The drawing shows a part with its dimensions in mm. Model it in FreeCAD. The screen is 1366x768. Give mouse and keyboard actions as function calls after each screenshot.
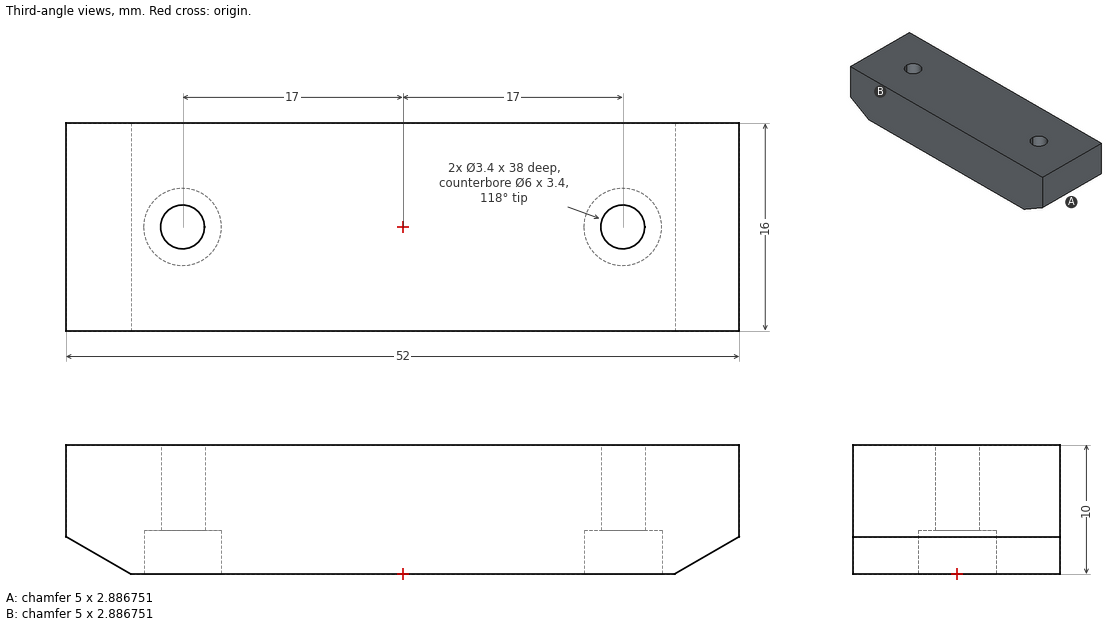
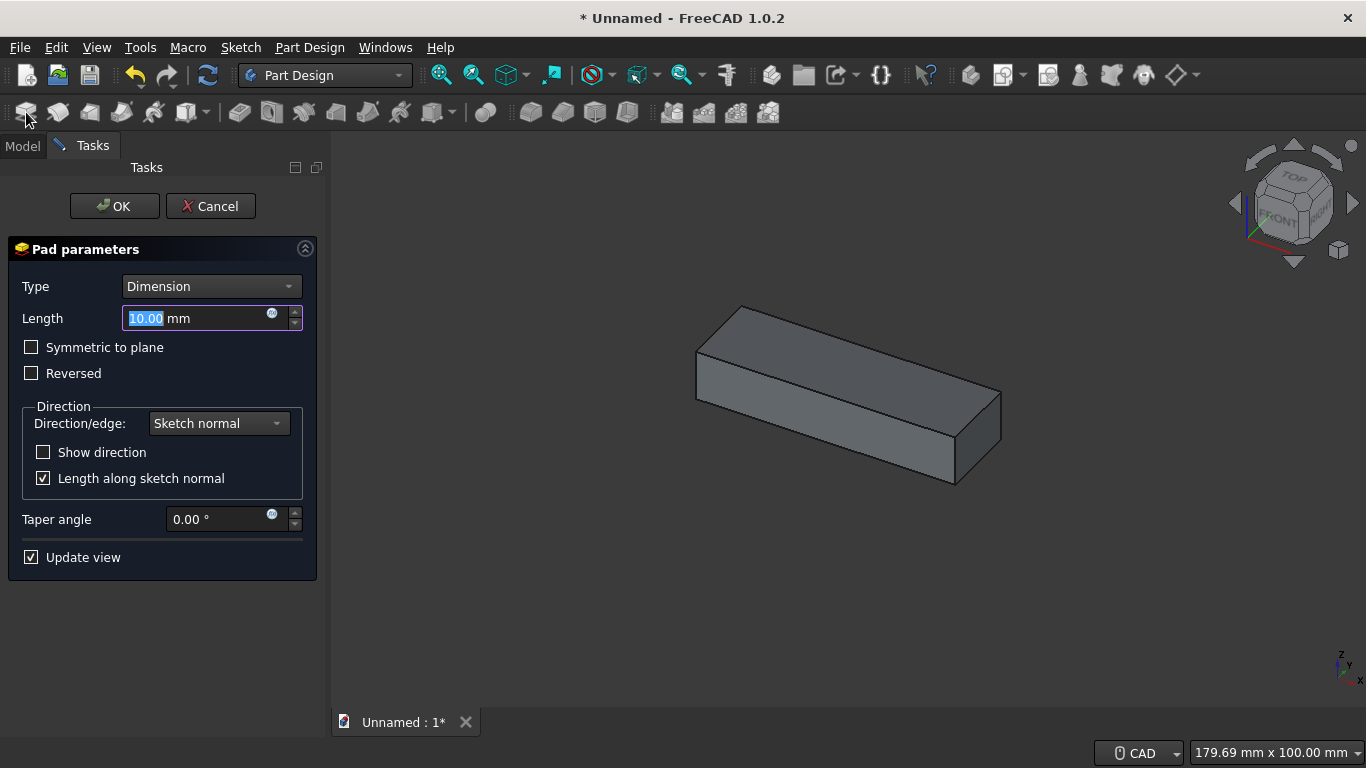
text(10)
key(Tab)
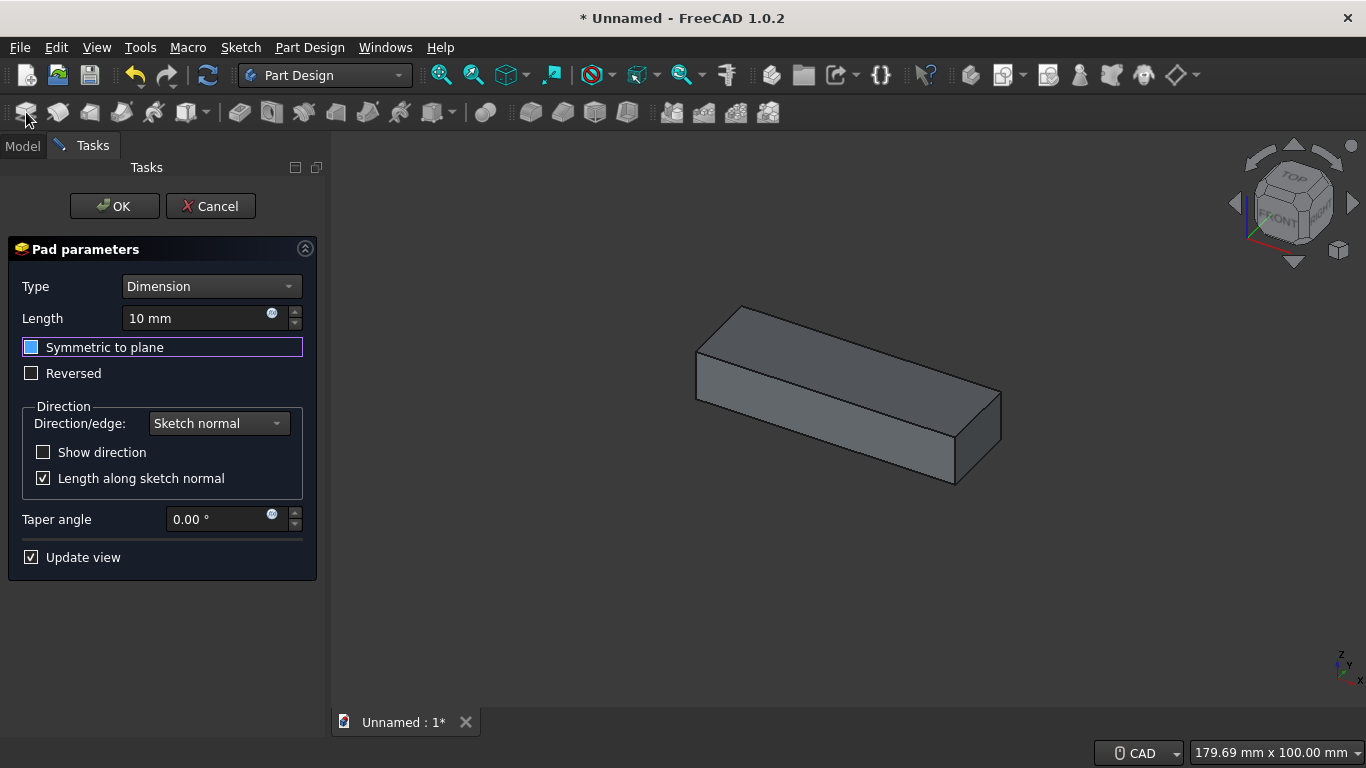
click(115, 206)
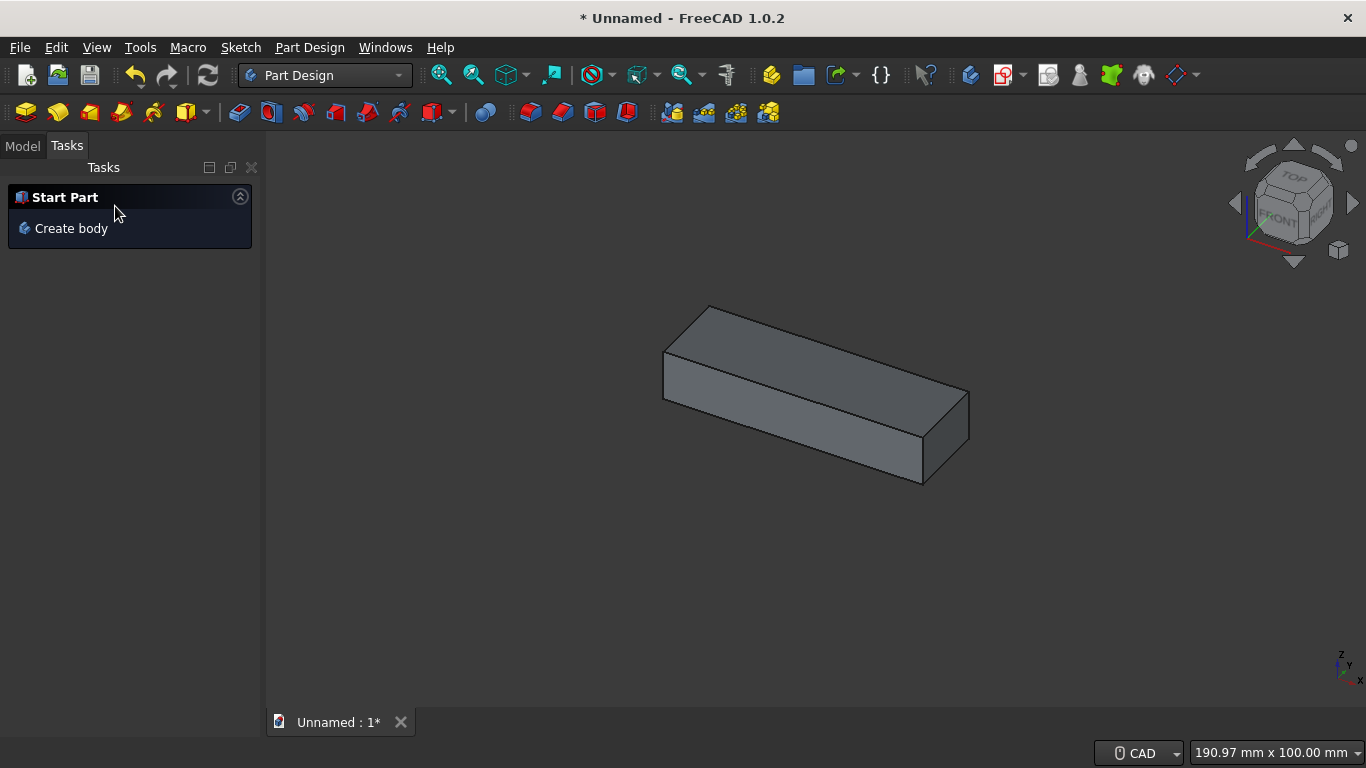
click(442, 76)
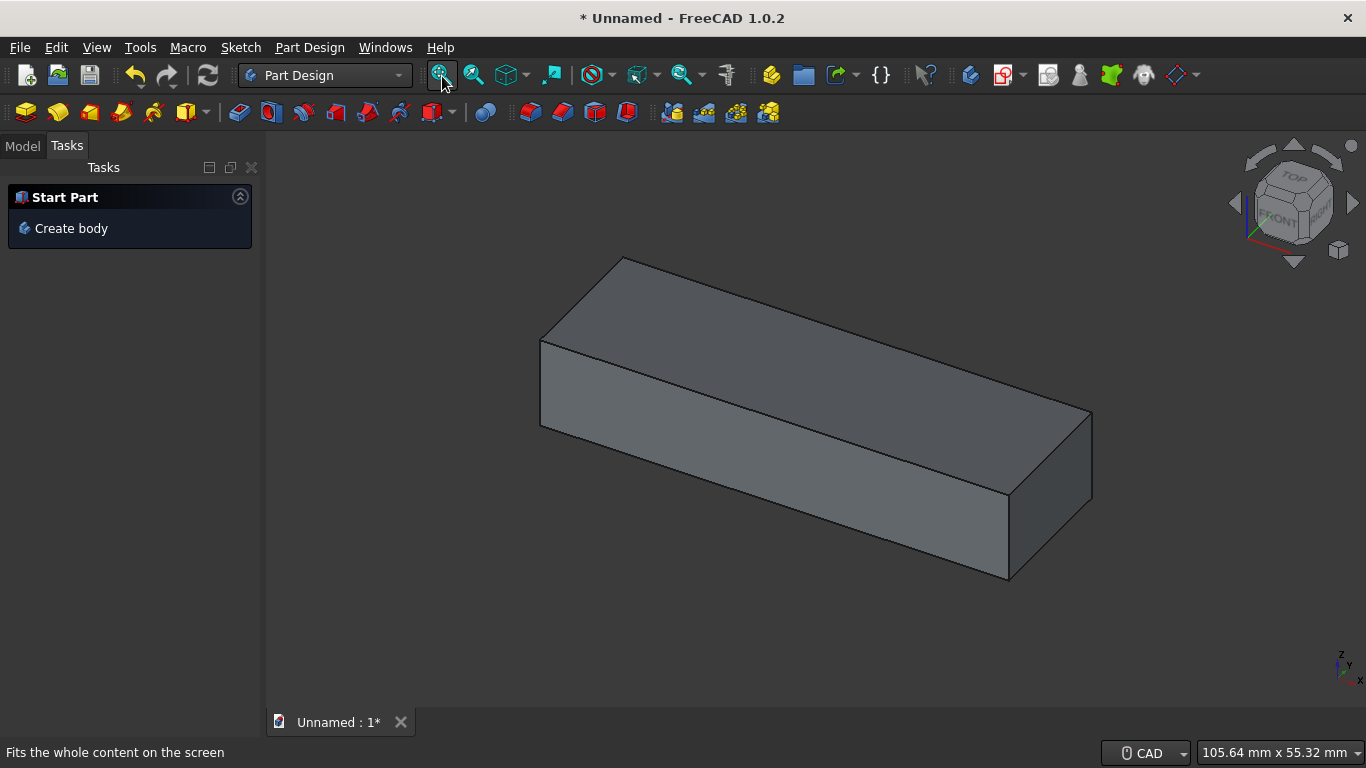
key(5)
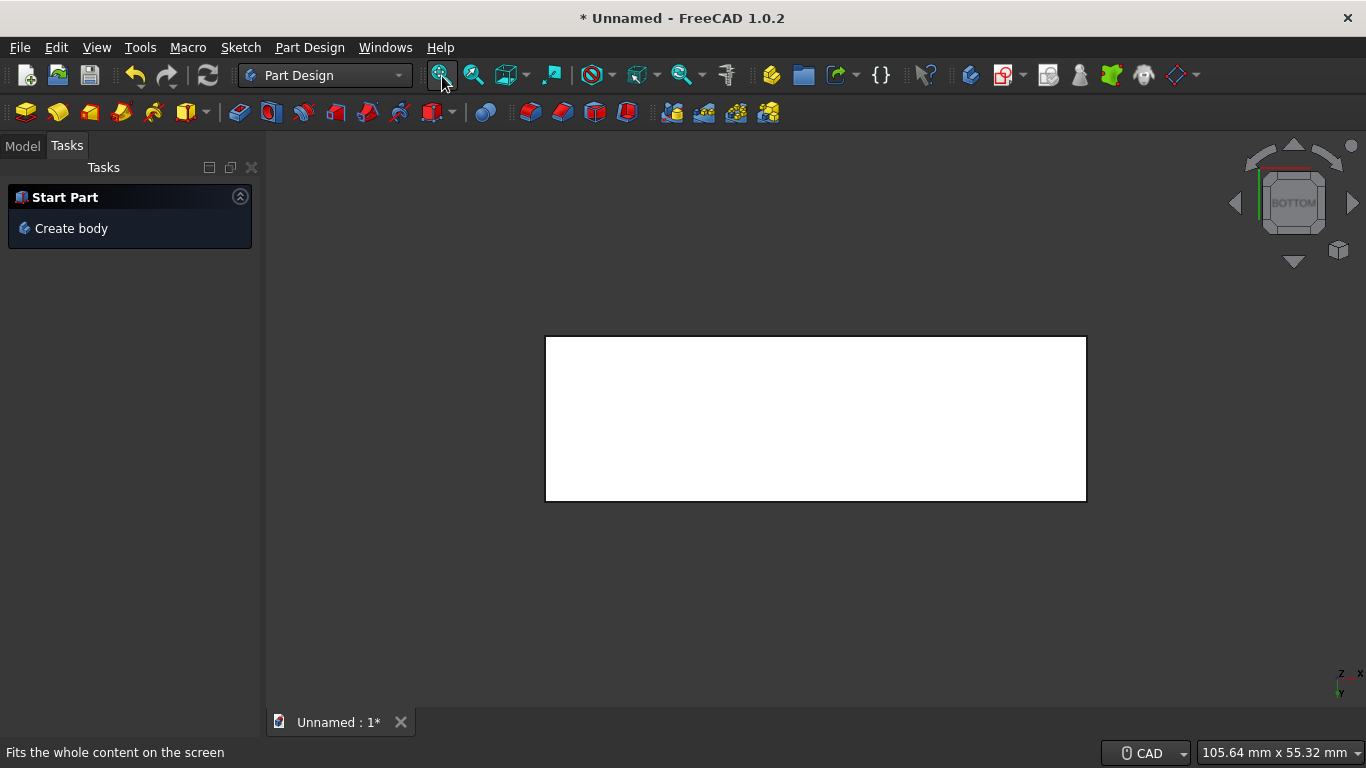
click(971, 418)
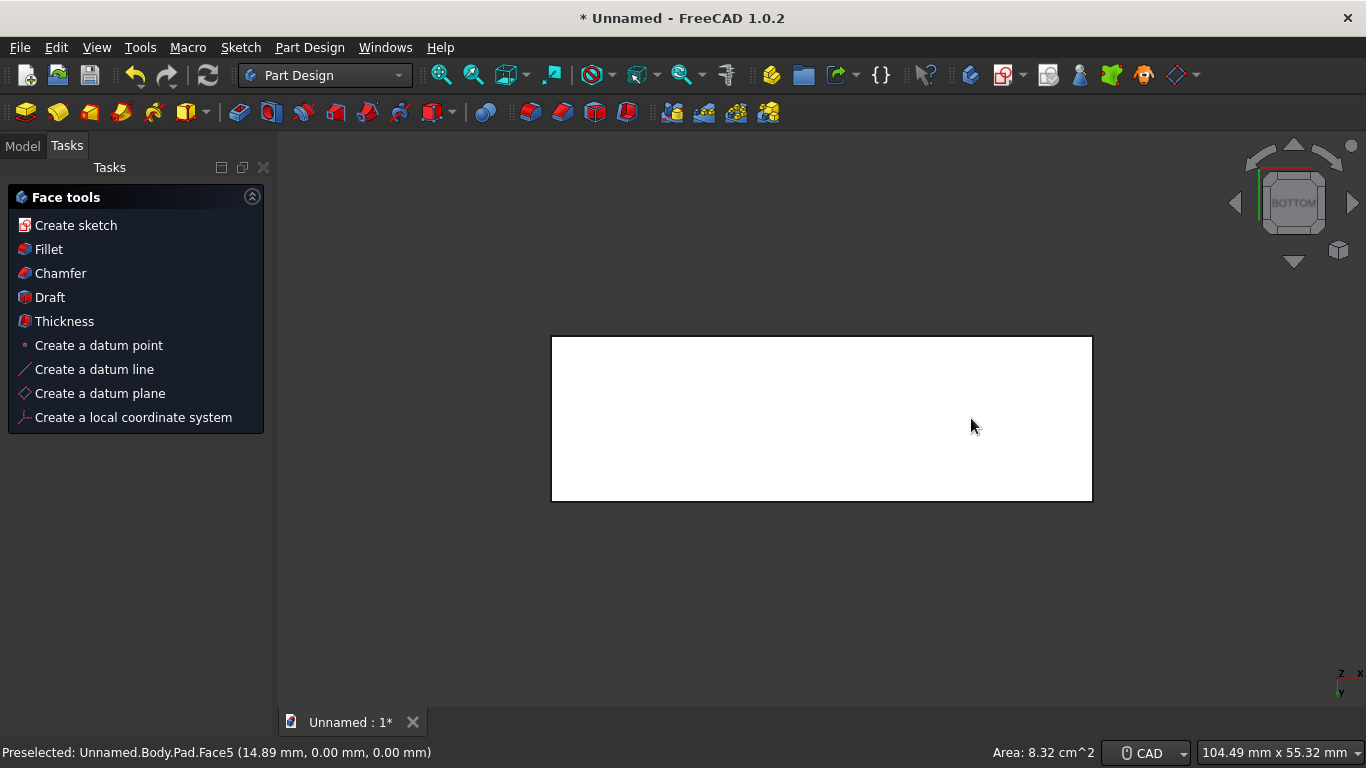
click(1004, 76)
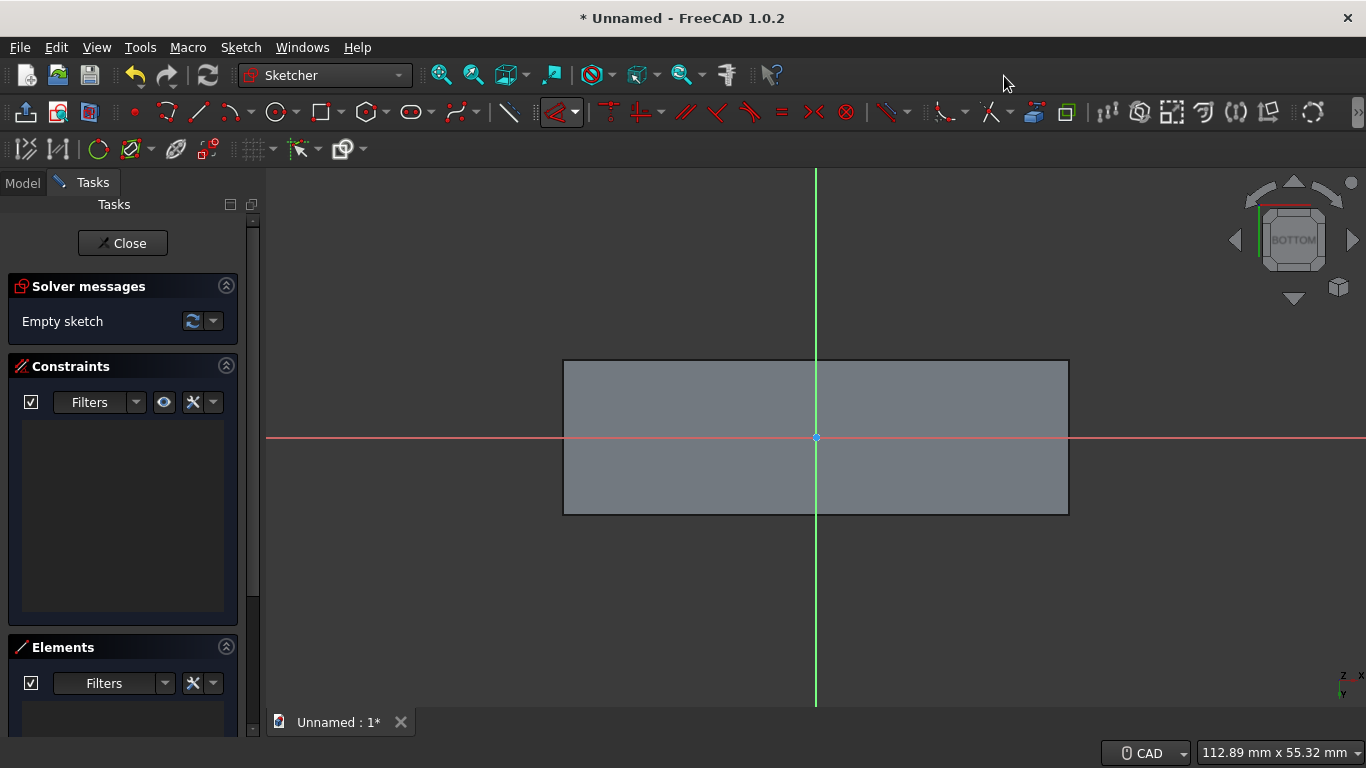
scroll(899, 438, up, 3)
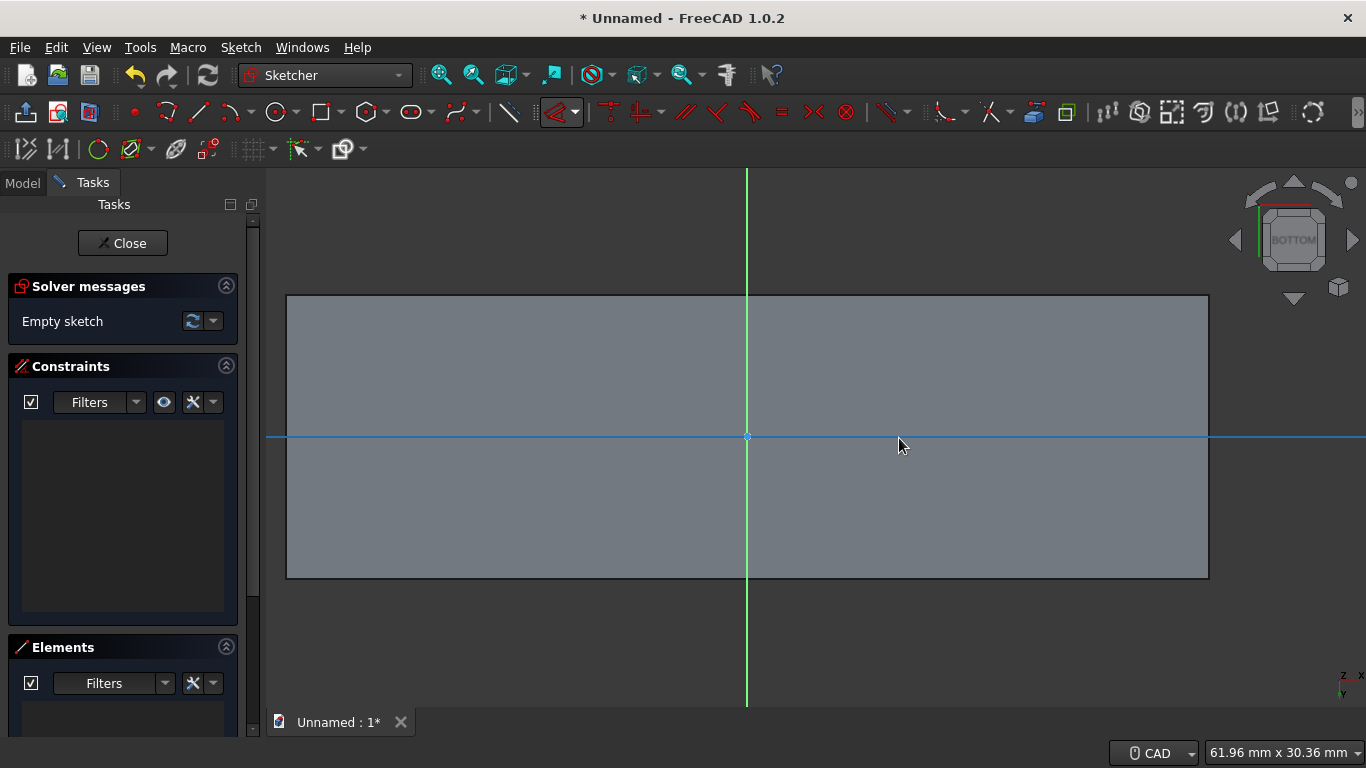
click(276, 112)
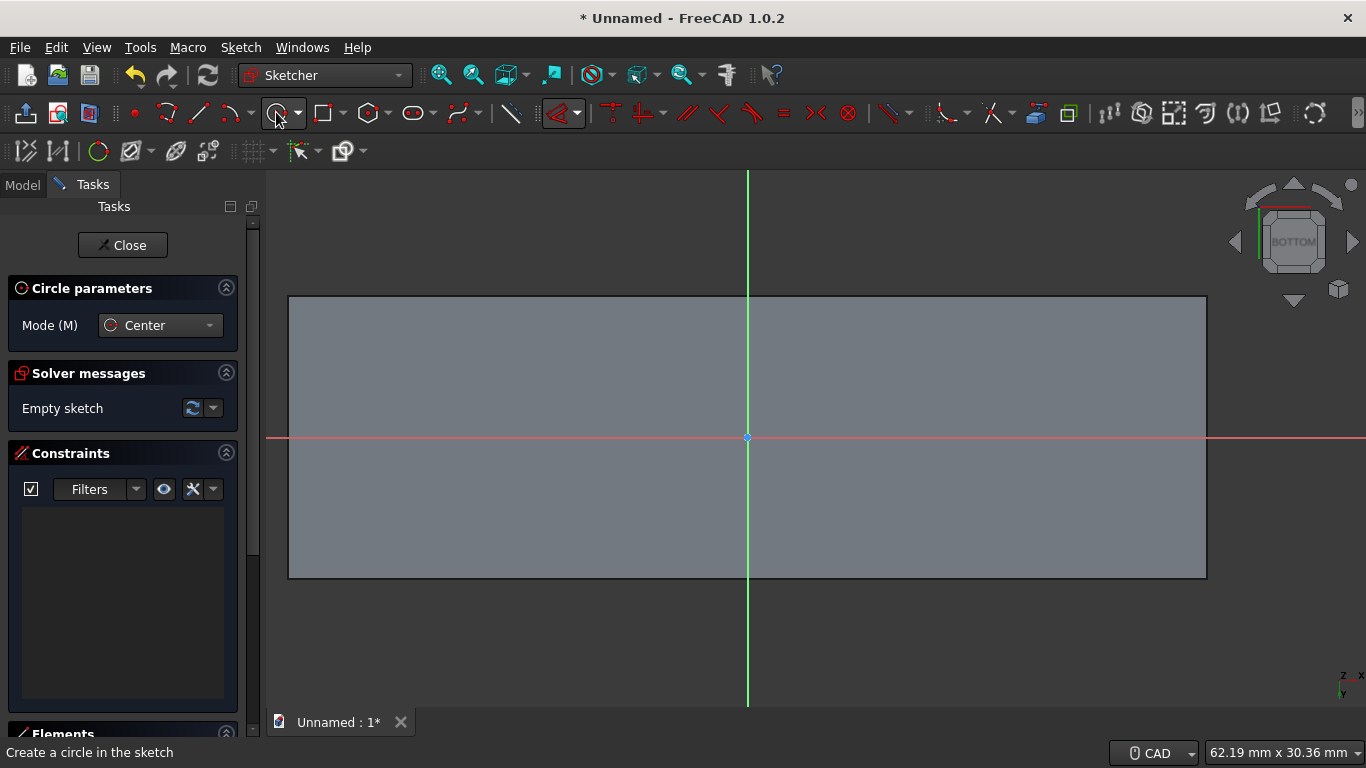
click(1048, 438)
move(1070, 416)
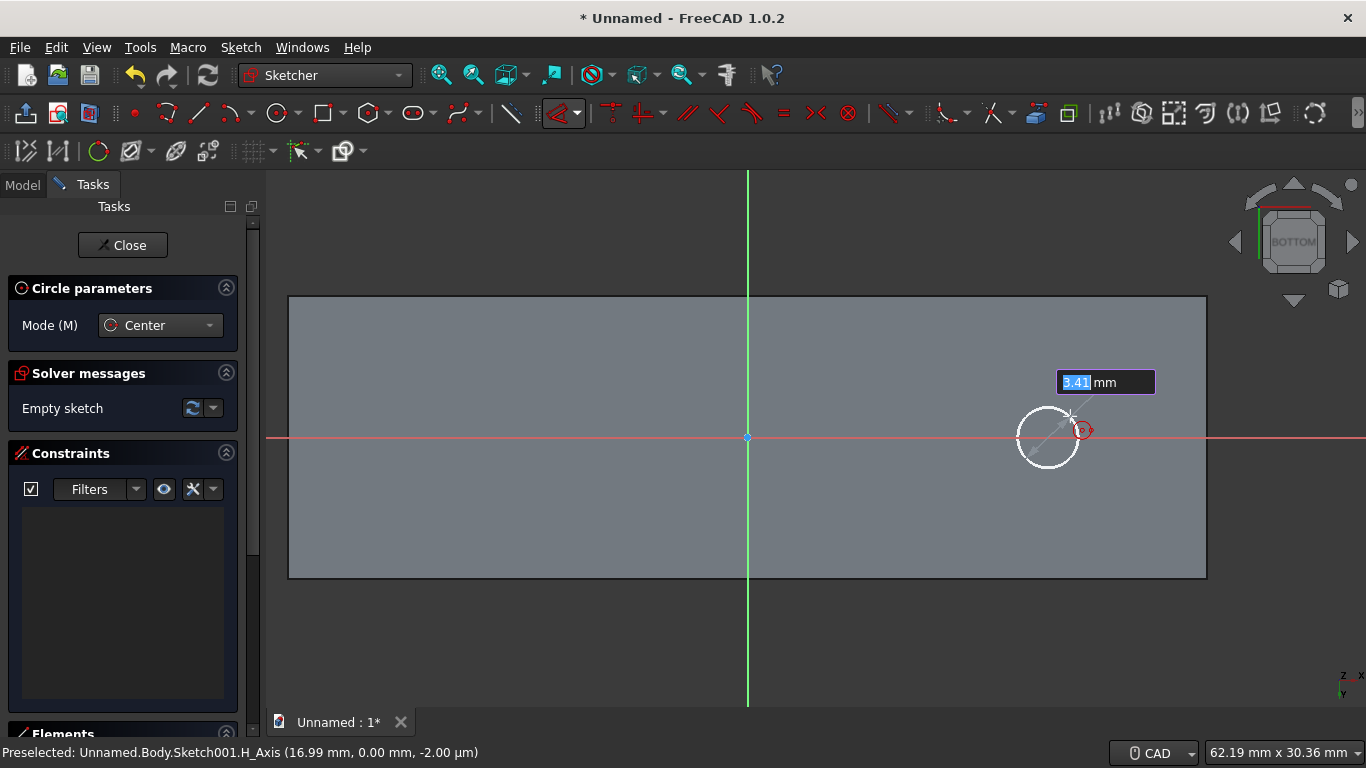
text(3.4)
key(Return)